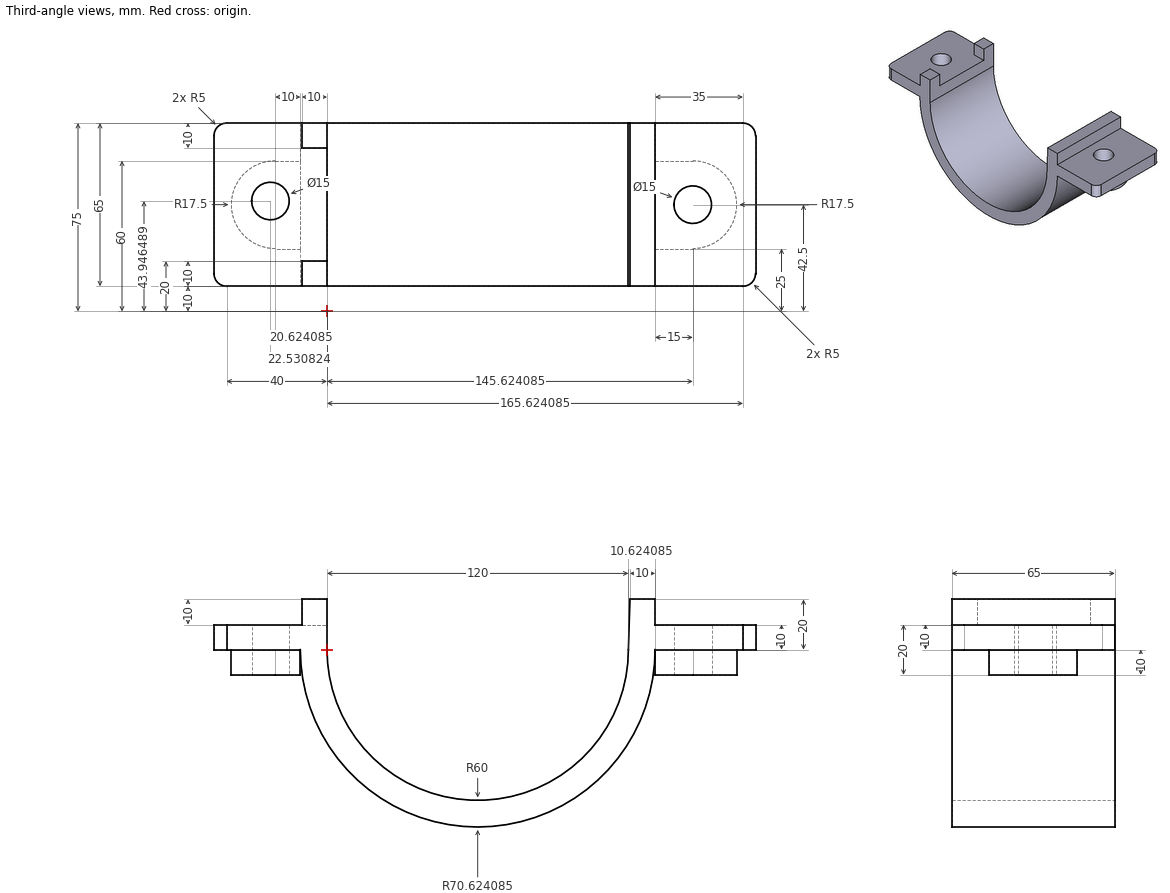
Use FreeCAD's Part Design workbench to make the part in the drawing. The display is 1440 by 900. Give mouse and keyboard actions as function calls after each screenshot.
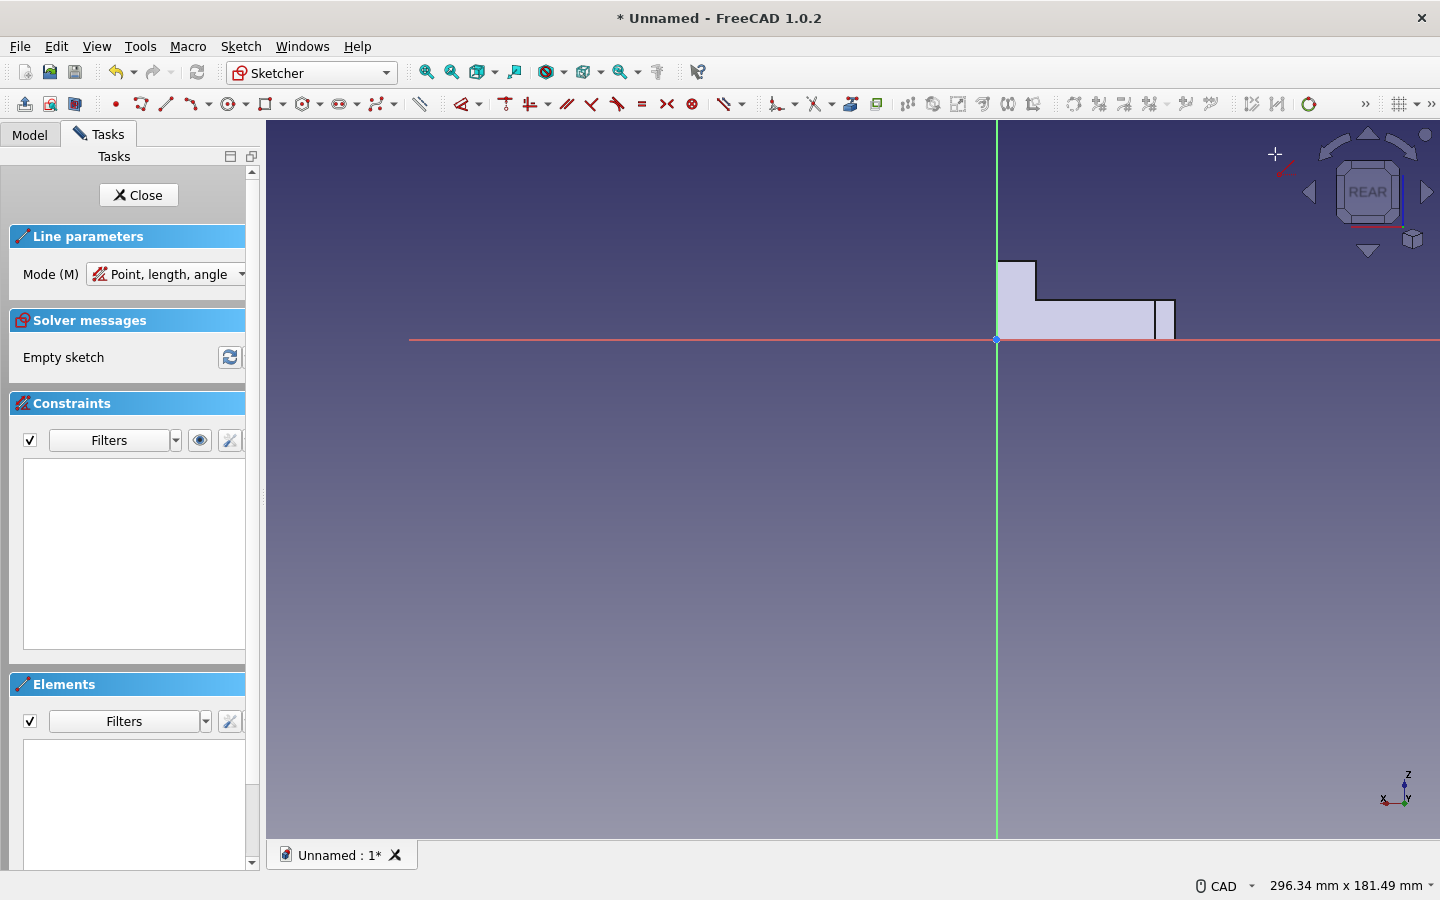
click(1039, 340)
click(997, 340)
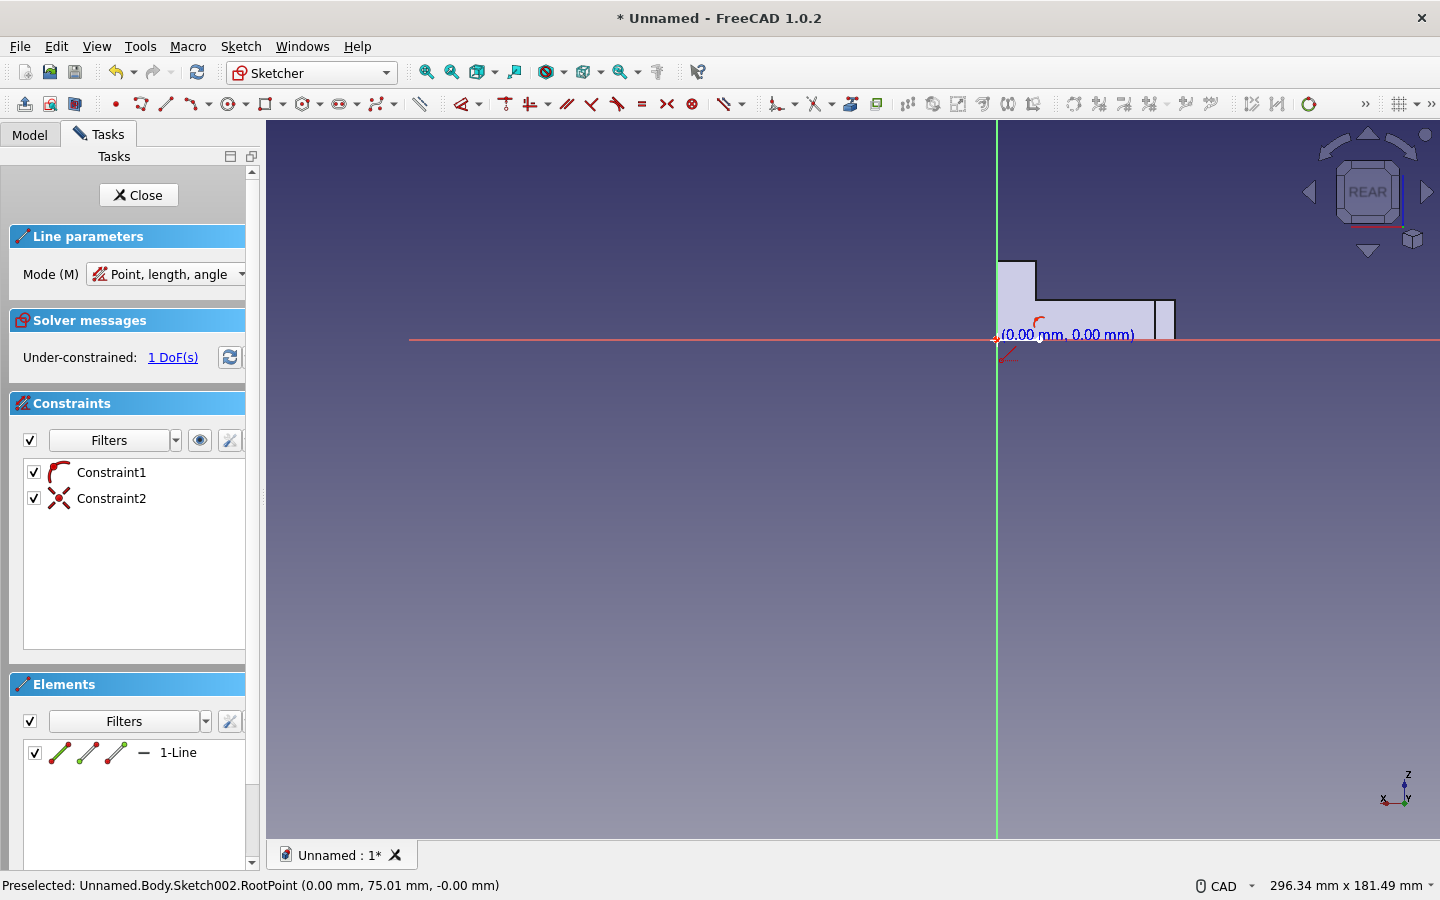
click(521, 340)
click(479, 349)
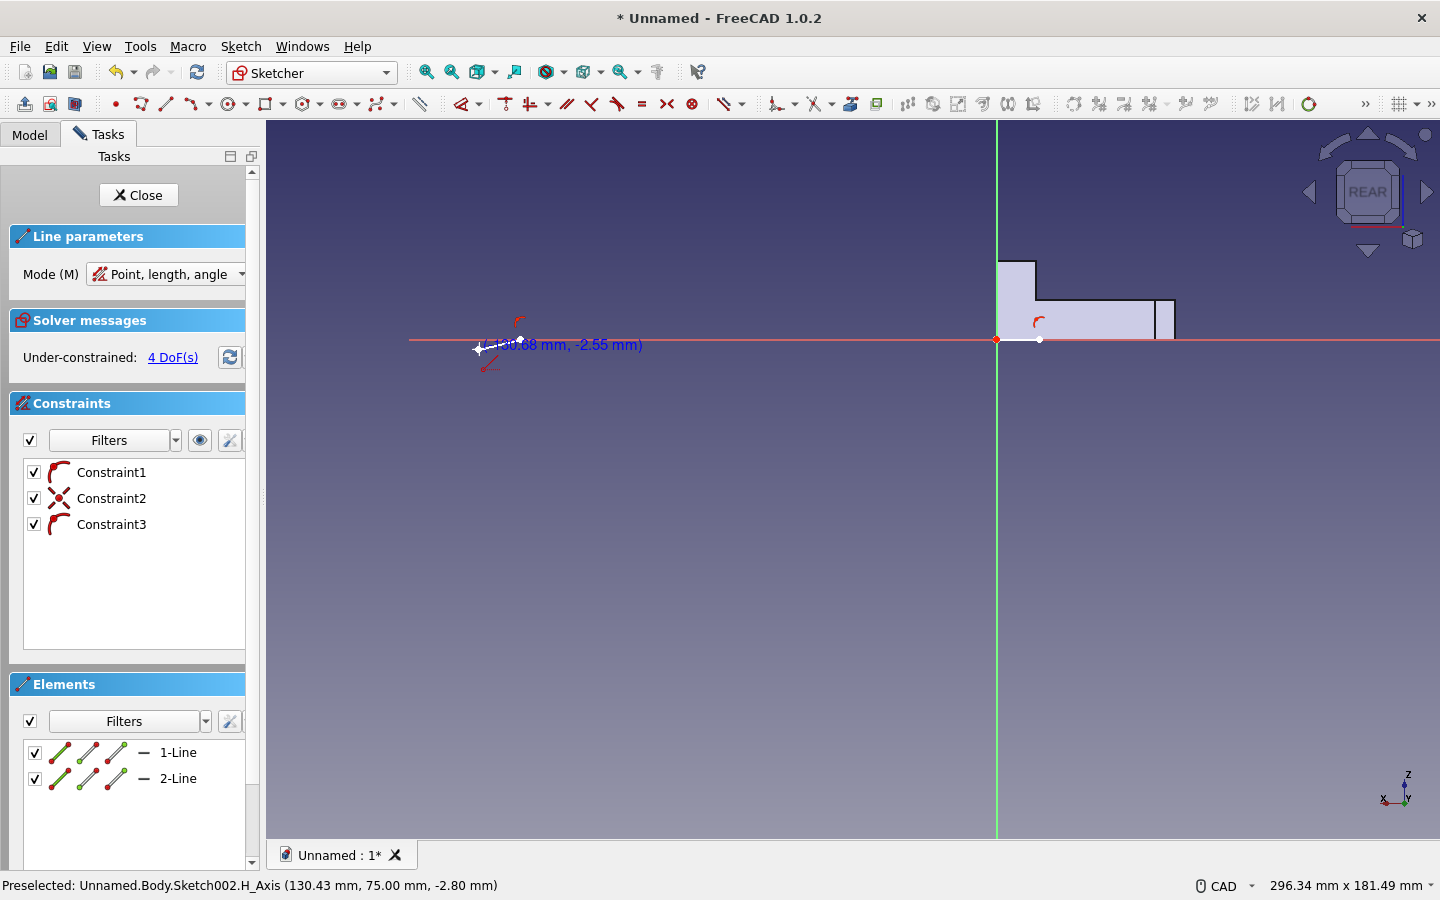
key(g)
key(3)
key(a)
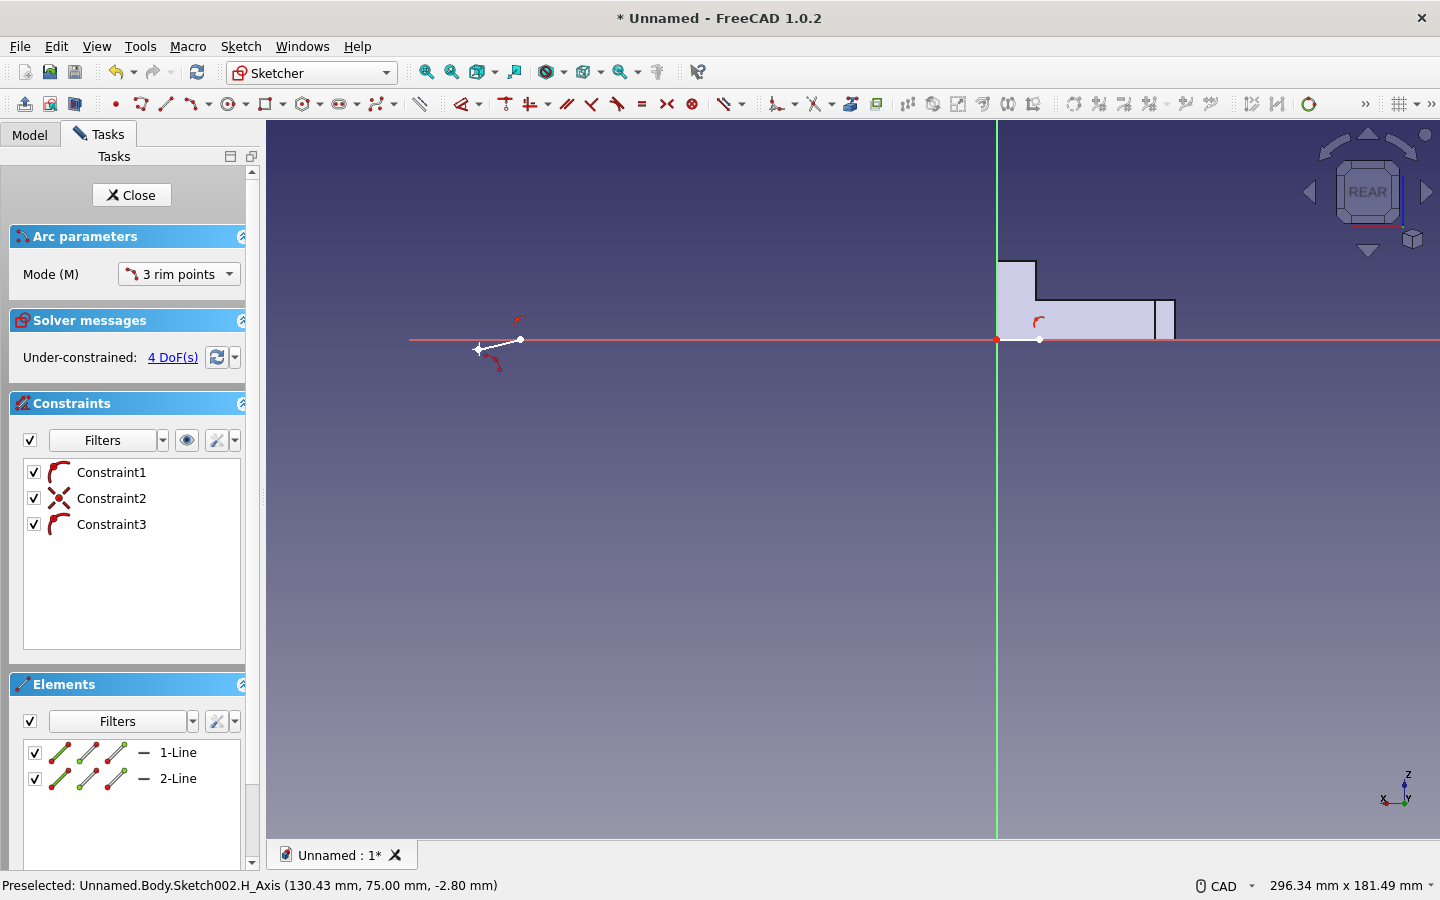
click(997, 340)
click(521, 340)
click(759, 578)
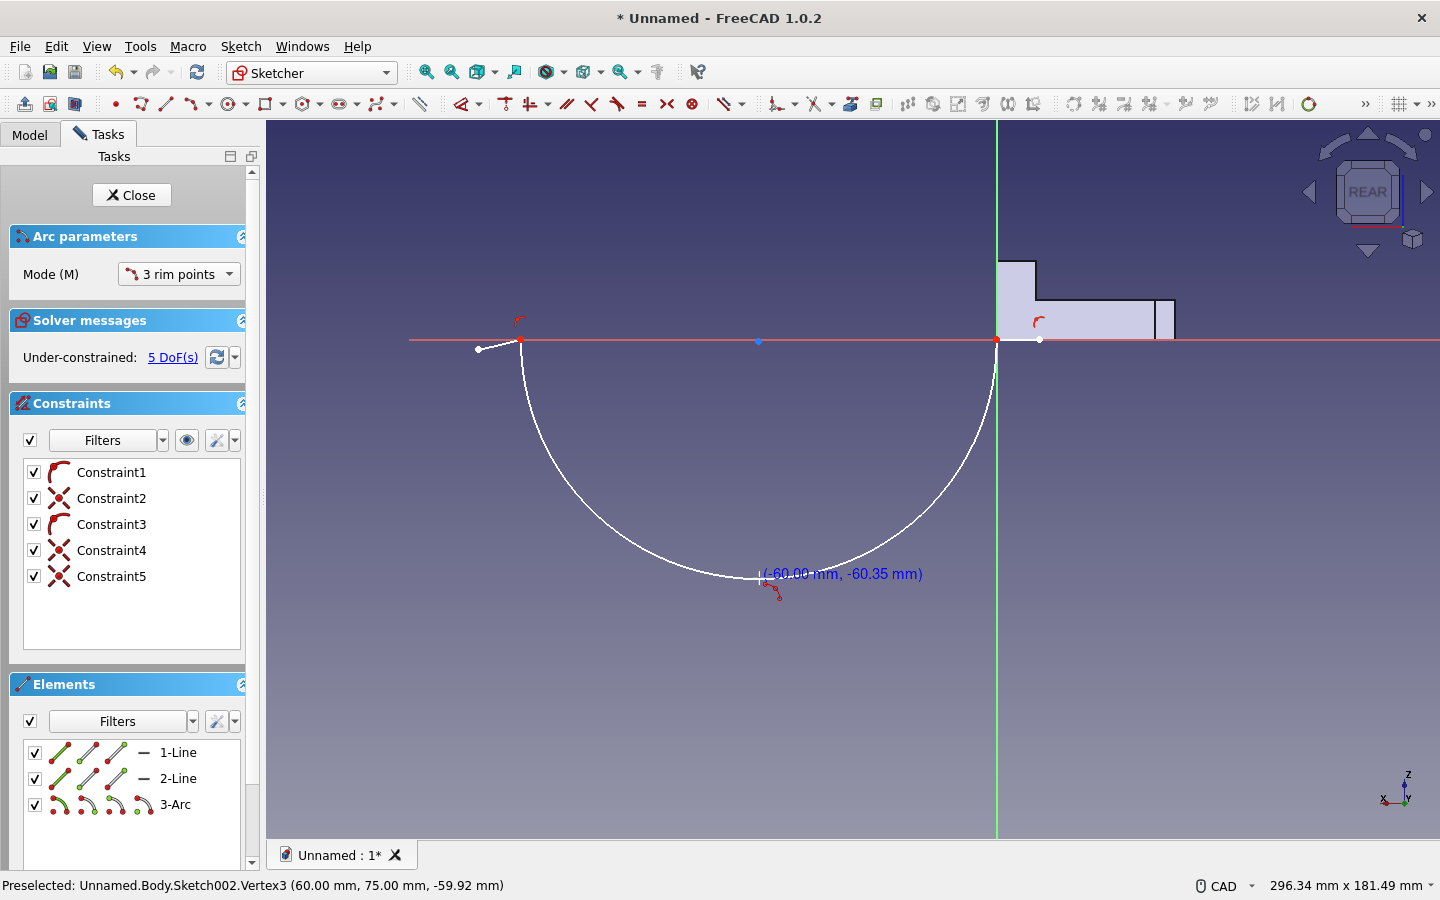
click(479, 350)
click(1039, 340)
click(759, 620)
key(Escape)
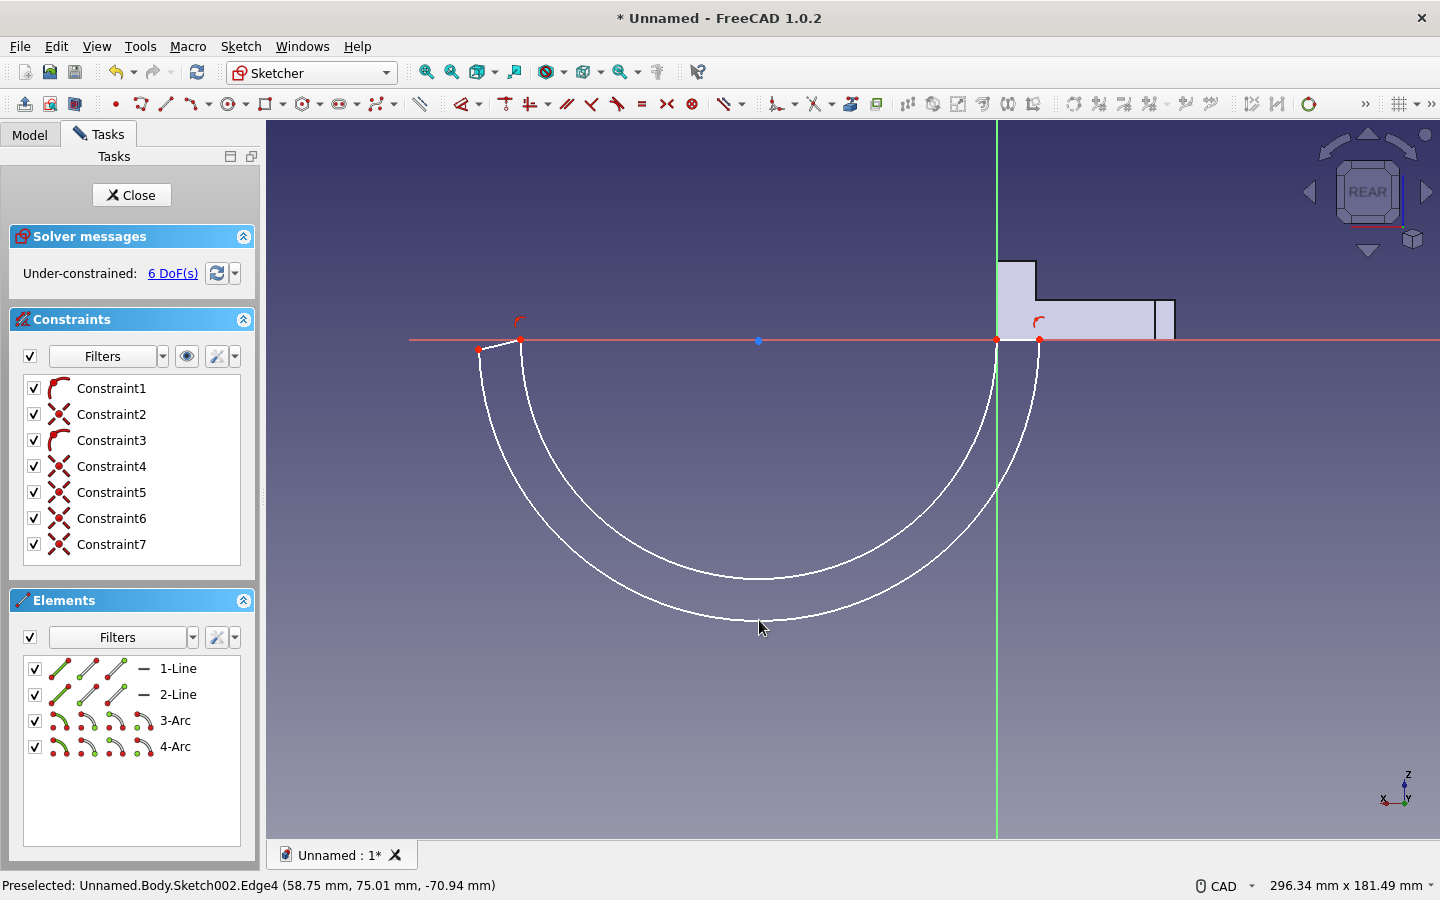
click(508, 343)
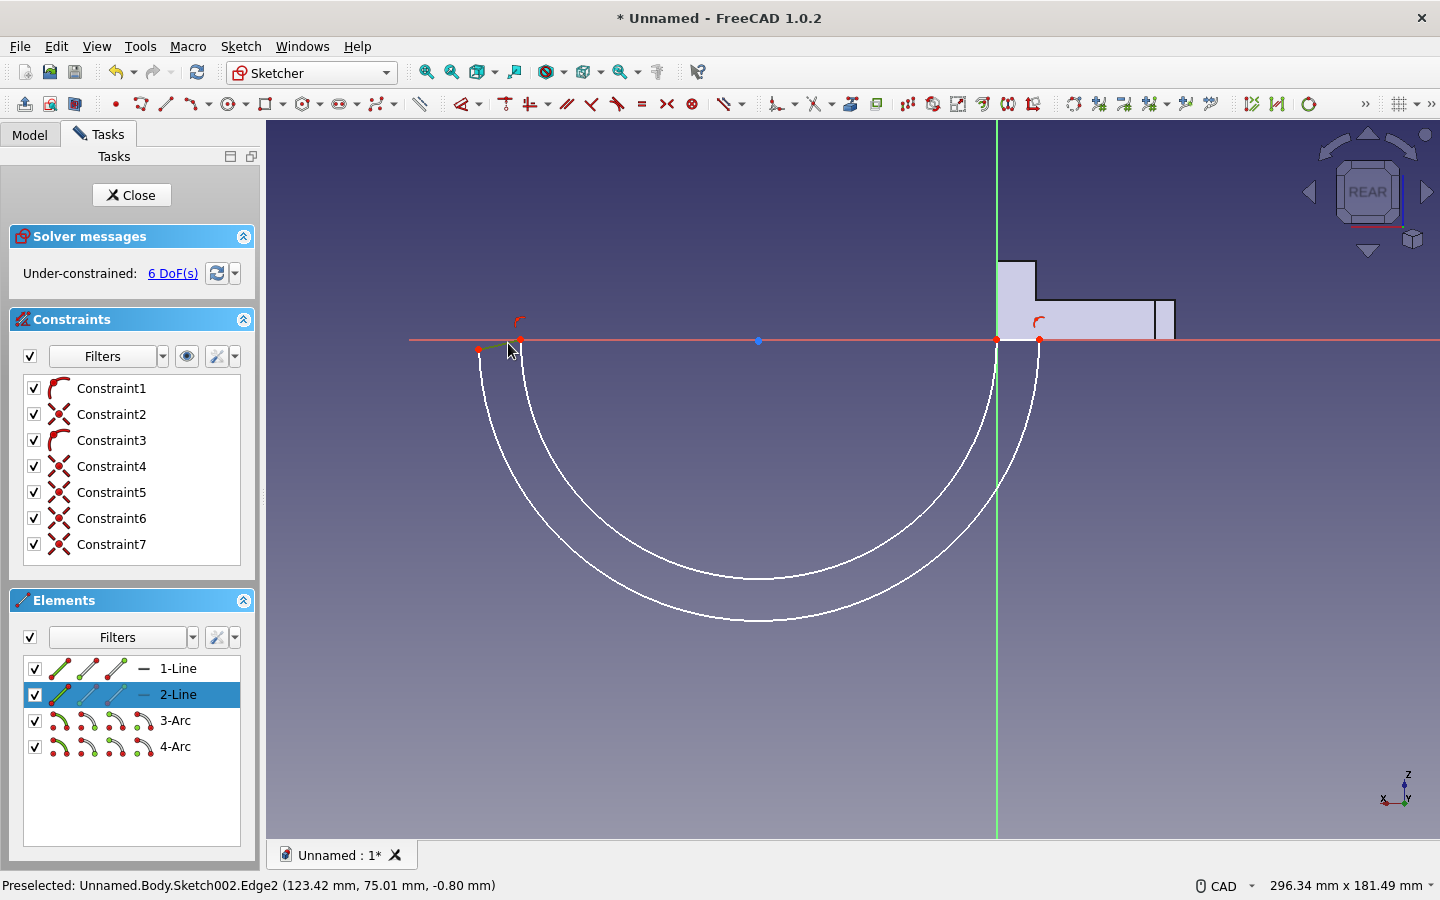
key(h)